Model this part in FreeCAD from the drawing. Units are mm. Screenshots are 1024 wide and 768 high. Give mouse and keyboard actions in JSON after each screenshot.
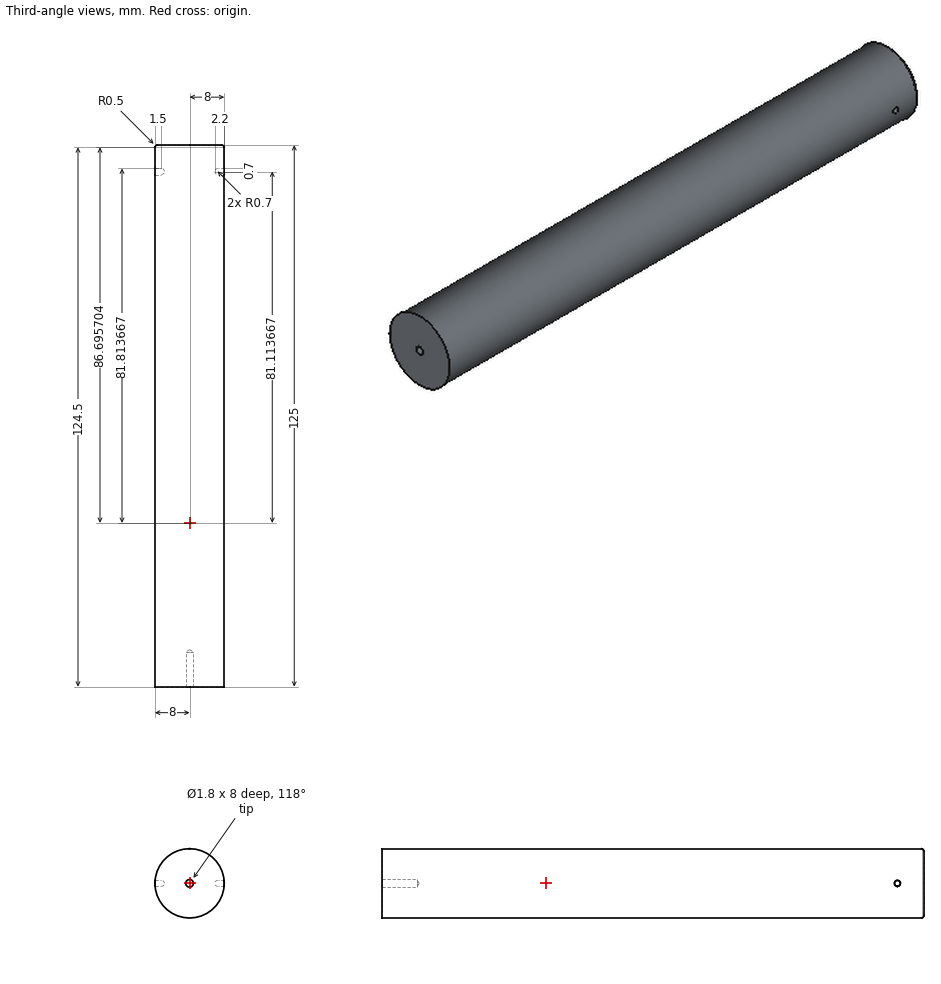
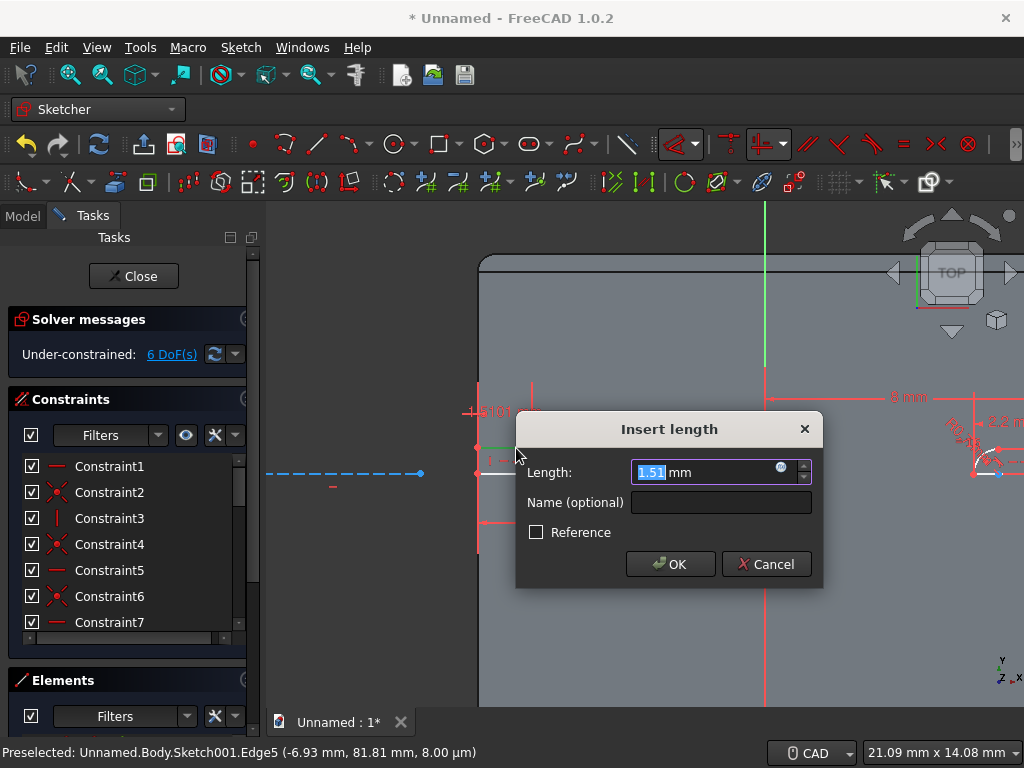
{"action": "type", "text": "1.5"}
{"action": "key", "text": "Return"}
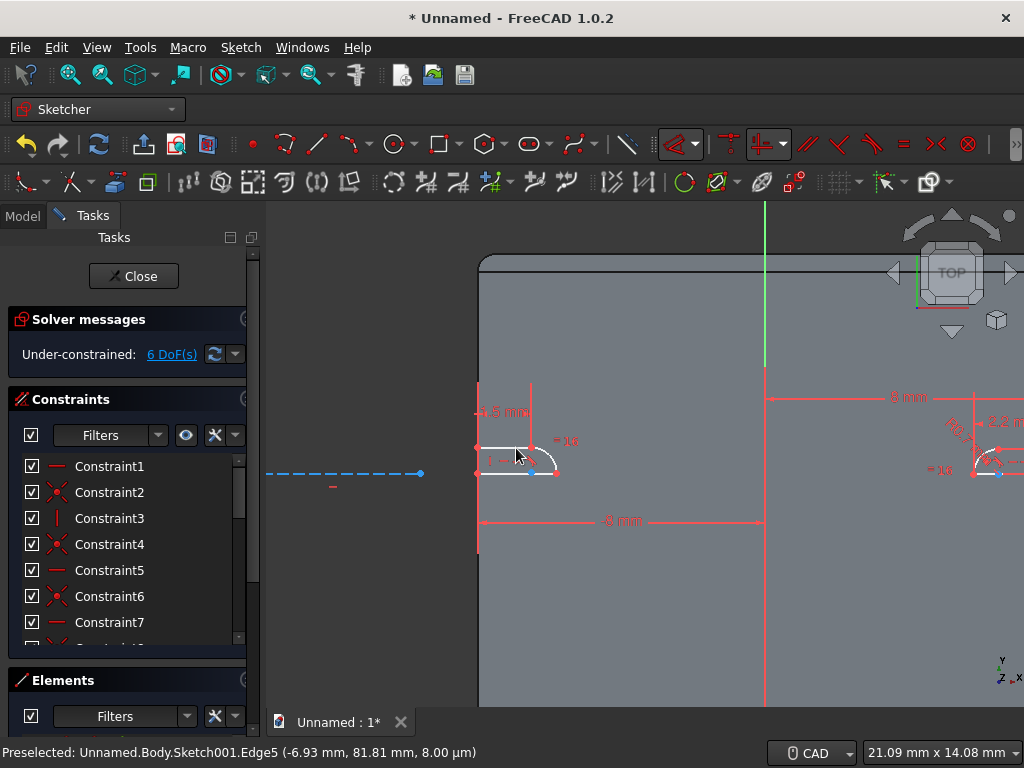
{"action": "scroll", "coordinate": [478, 458], "scroll_direction": "up", "scroll_amount": 3}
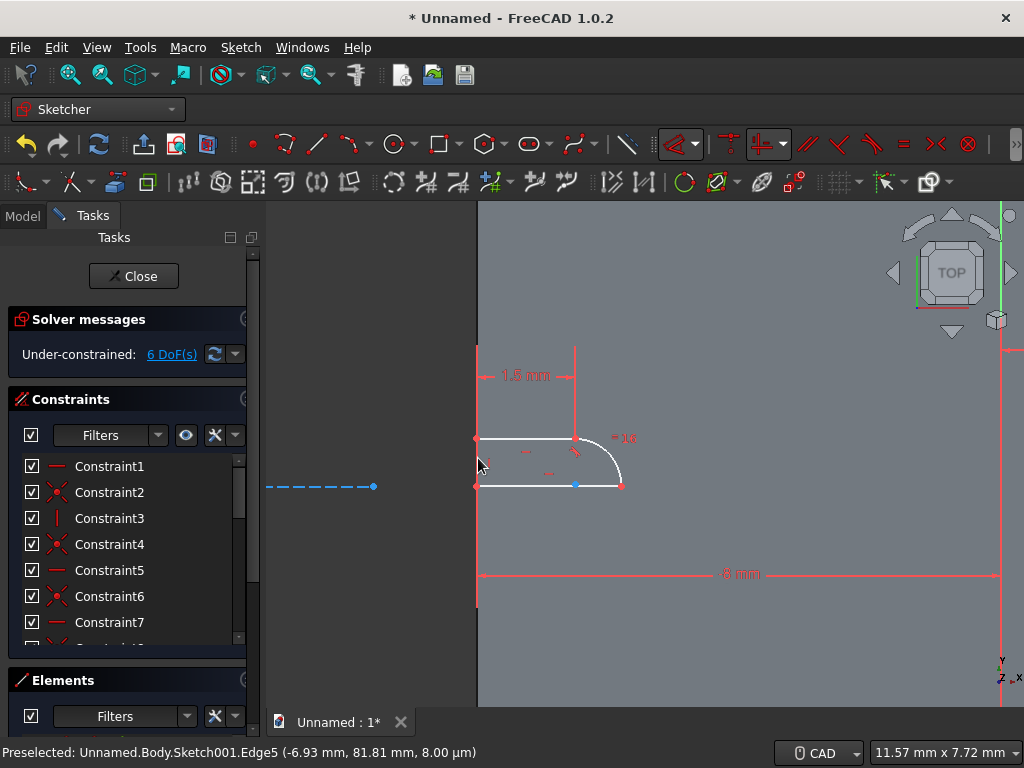
{"action": "left_click", "coordinate": [477, 458]}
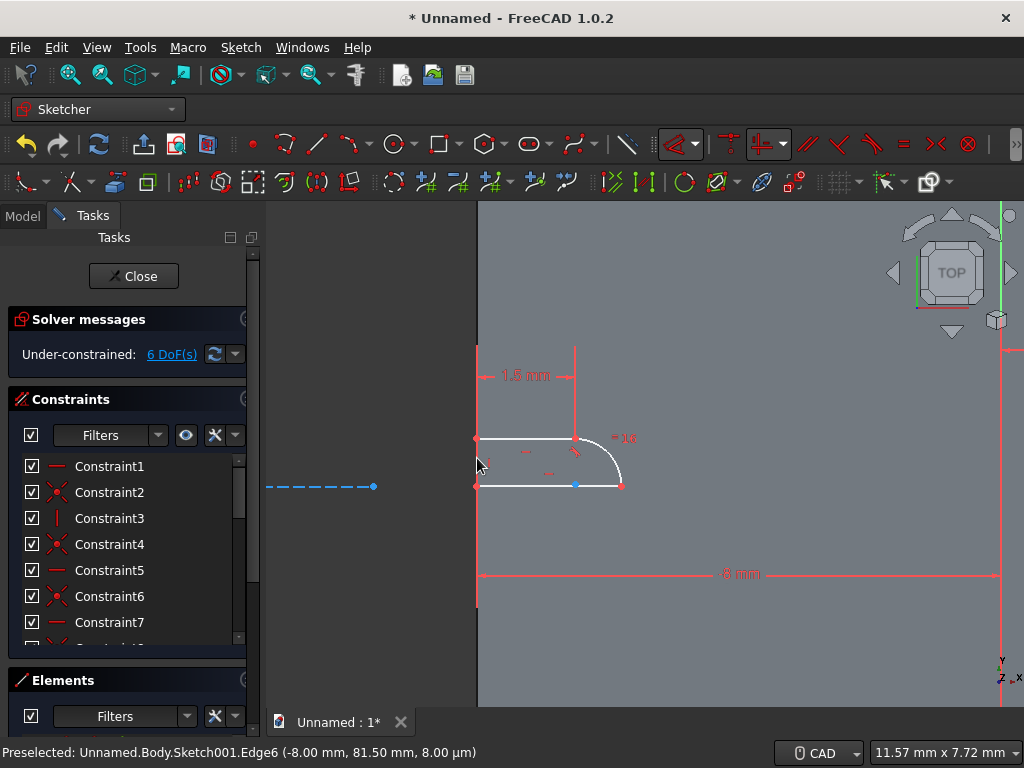
{"action": "key", "text": "i"}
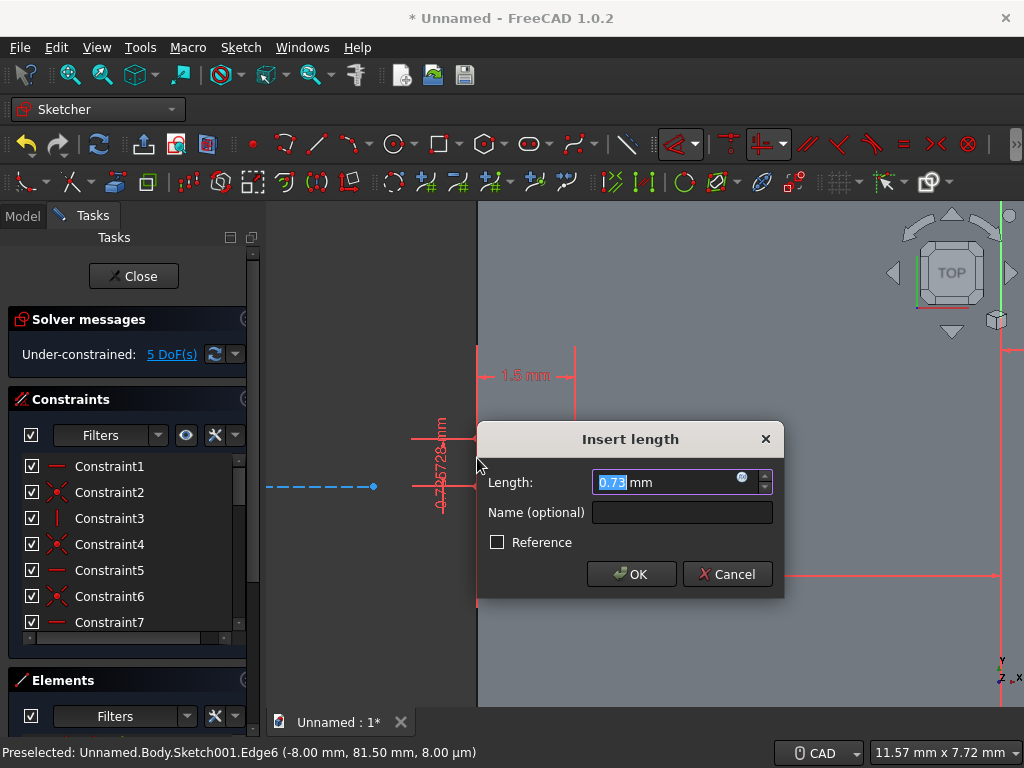
{"action": "type", "text": "0.7"}
{"action": "key", "text": "Return"}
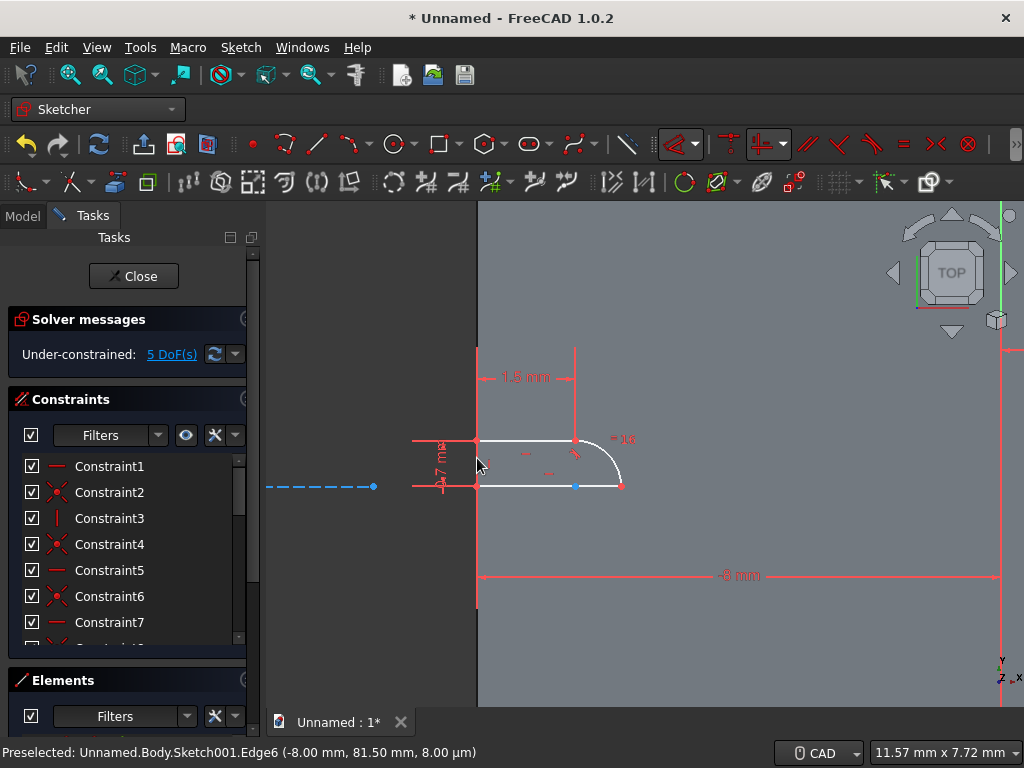
{"action": "scroll", "coordinate": [506, 452], "scroll_direction": "down", "scroll_amount": 7}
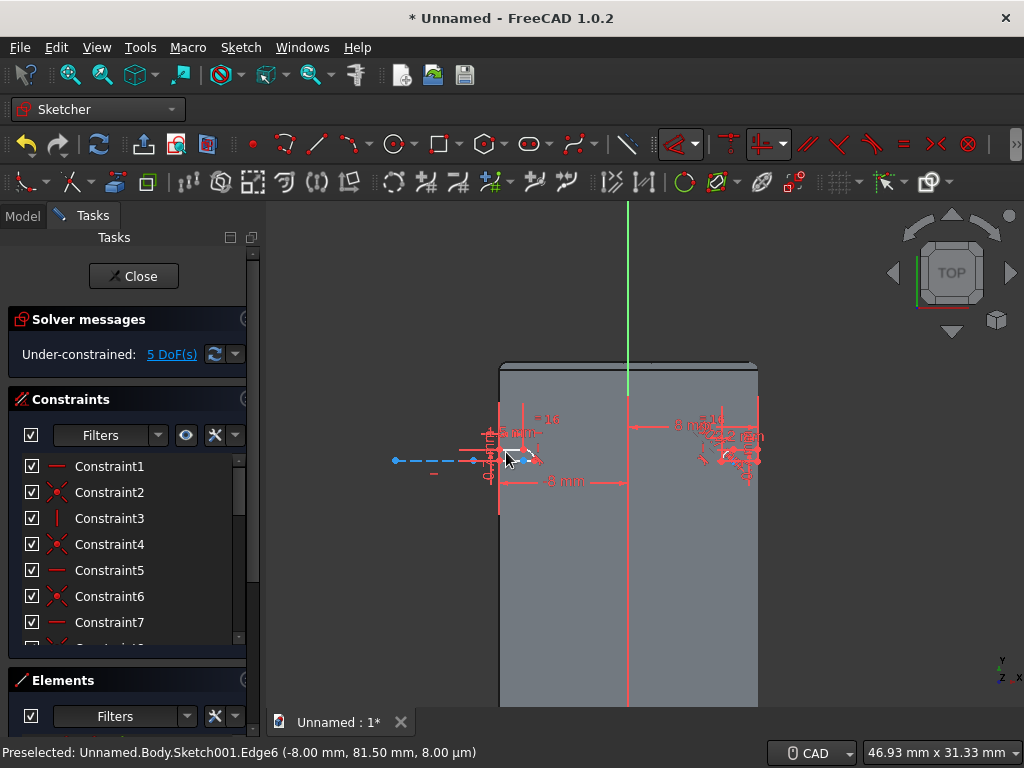
{"action": "left_click", "coordinate": [722, 461]}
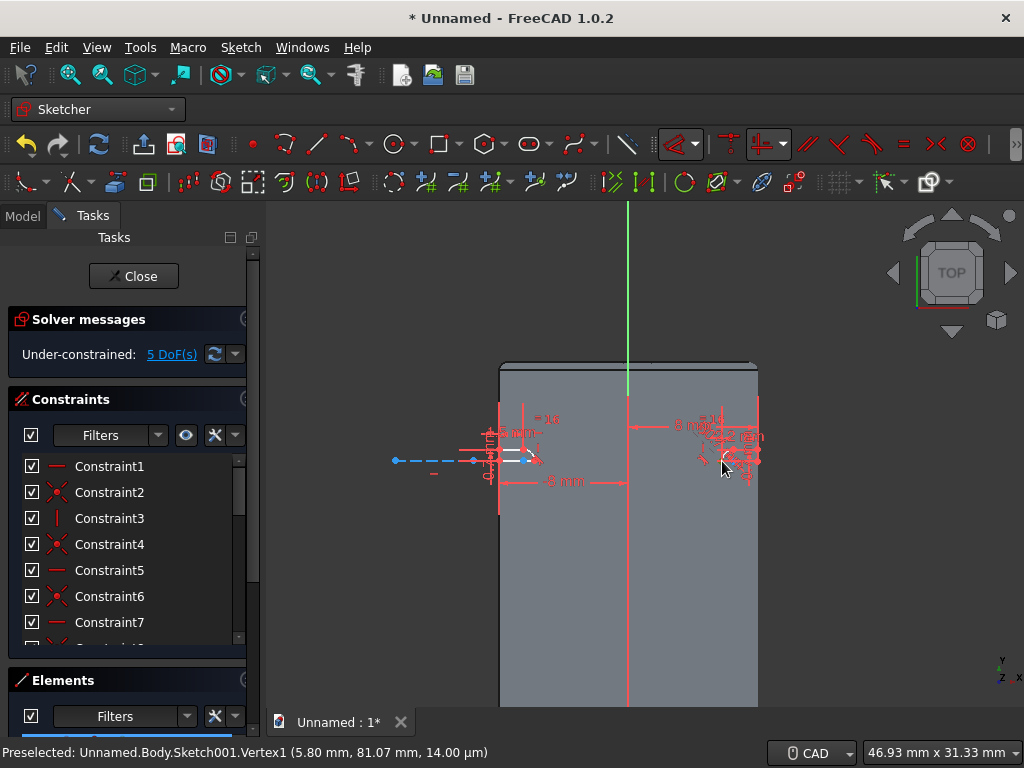
{"action": "key", "text": "i"}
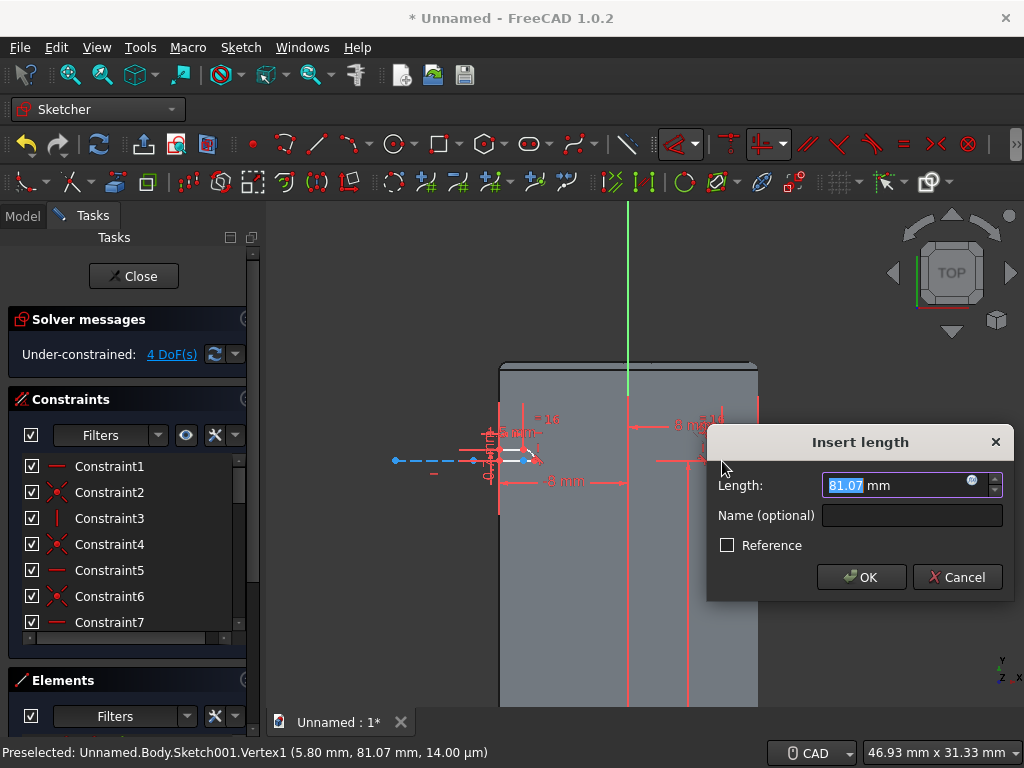
{"action": "type", "text": "81.113667"}
{"action": "key", "text": "Return"}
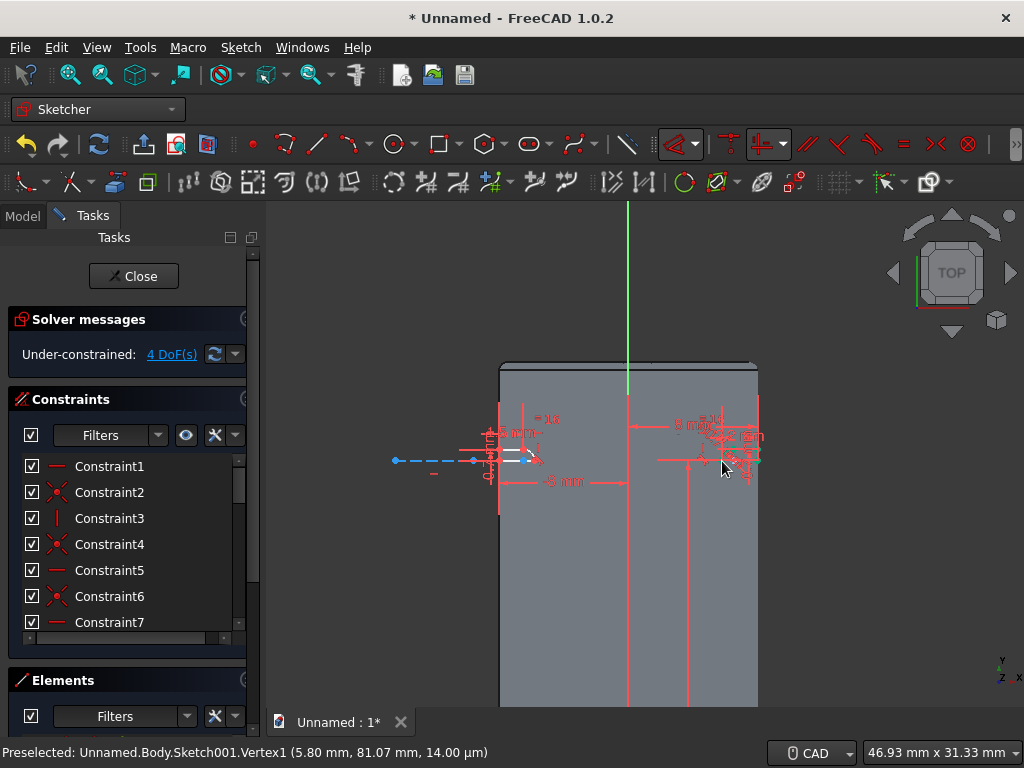
{"action": "left_click", "coordinate": [523, 450]}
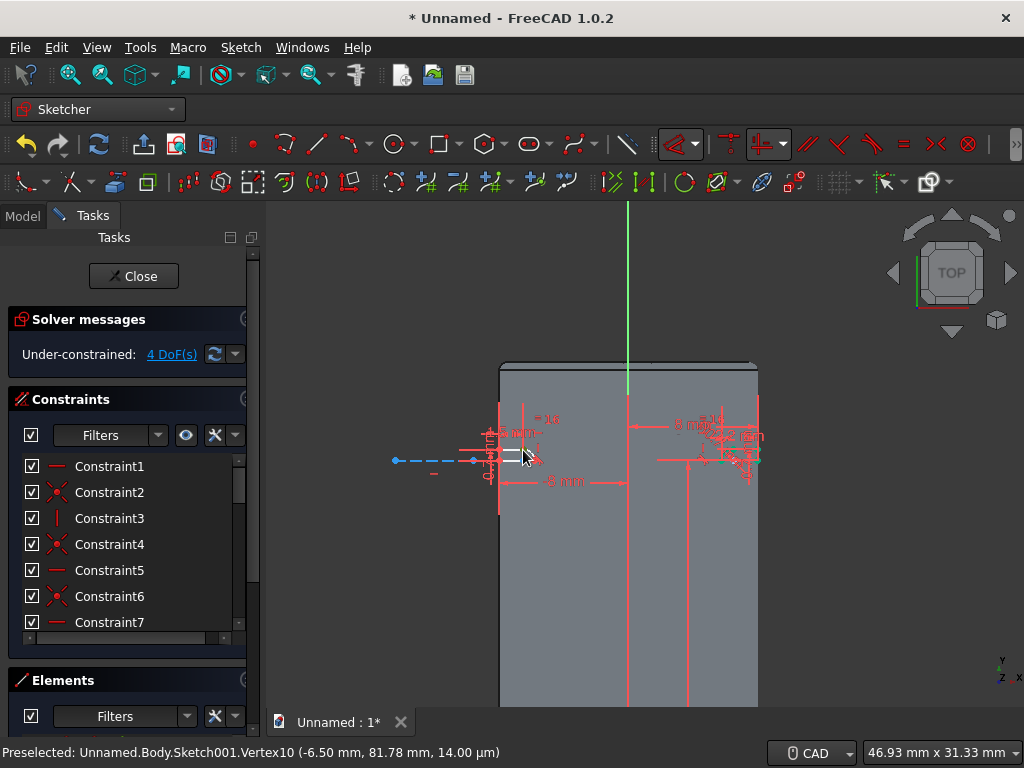
{"action": "key", "text": "i"}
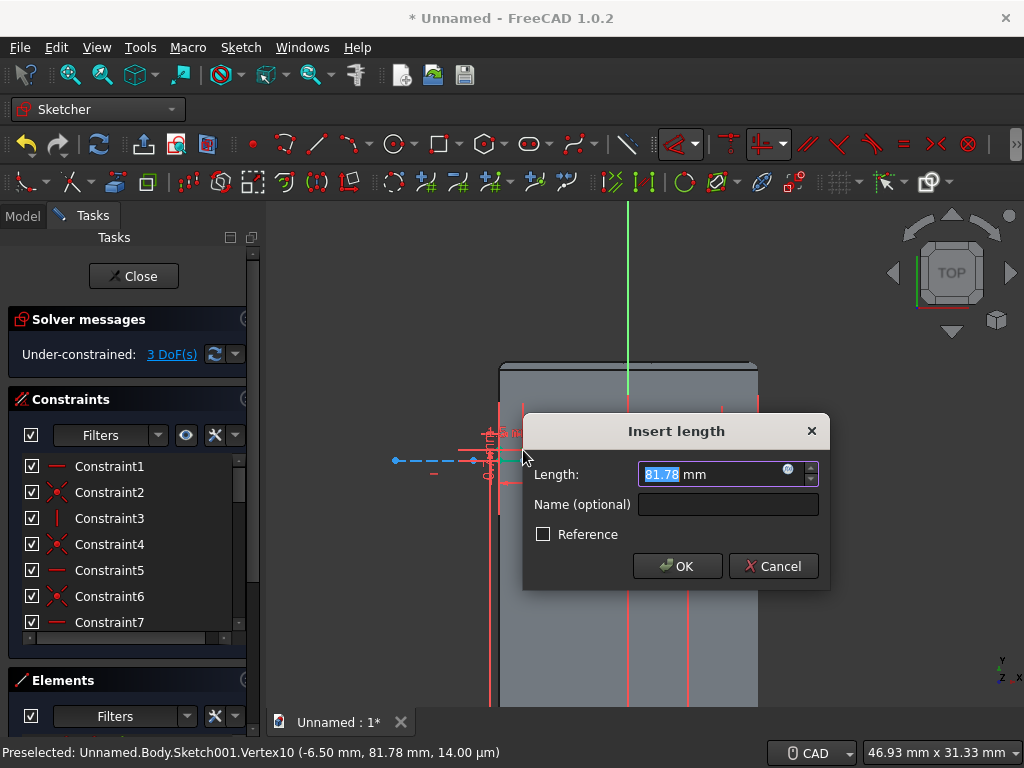
{"action": "type", "text": "81.813667"}
{"action": "key", "text": "Return"}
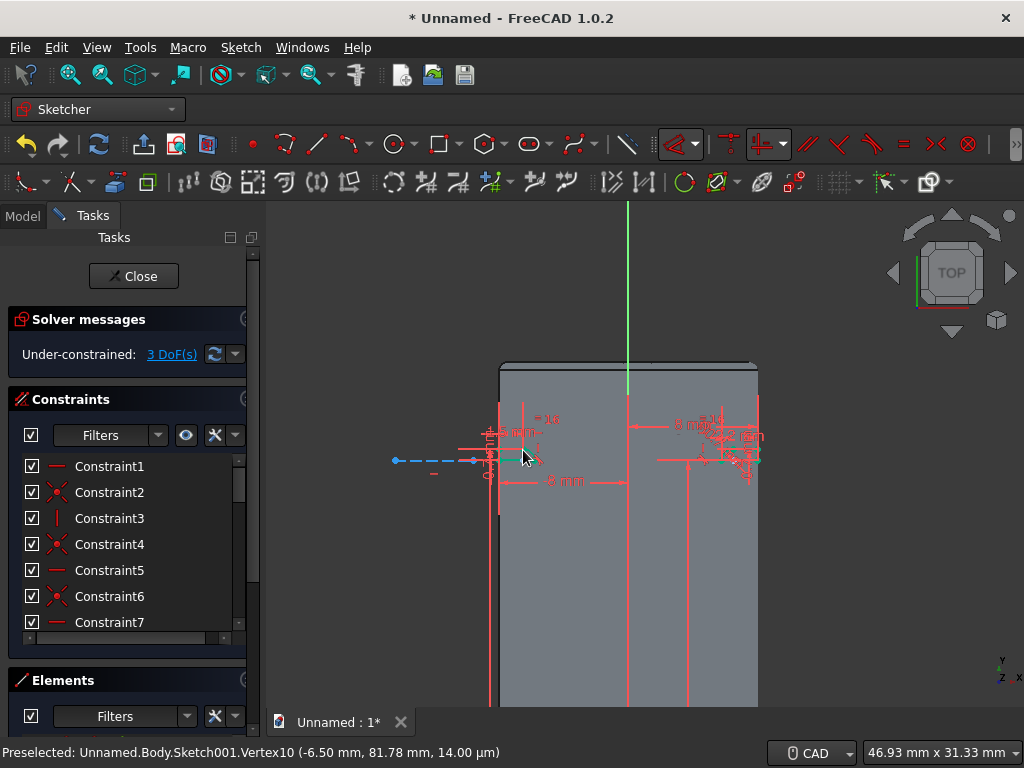
{"action": "left_click", "coordinate": [473, 461]}